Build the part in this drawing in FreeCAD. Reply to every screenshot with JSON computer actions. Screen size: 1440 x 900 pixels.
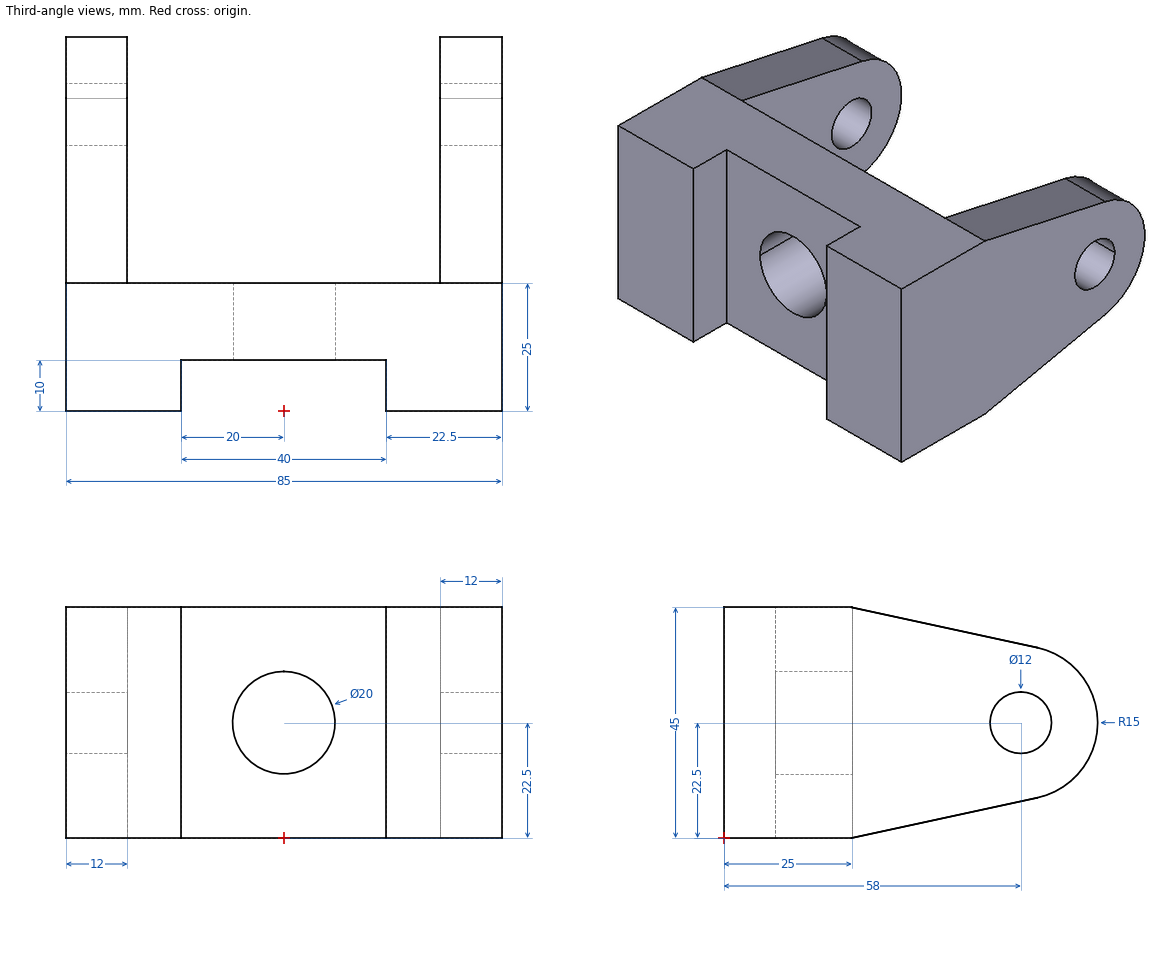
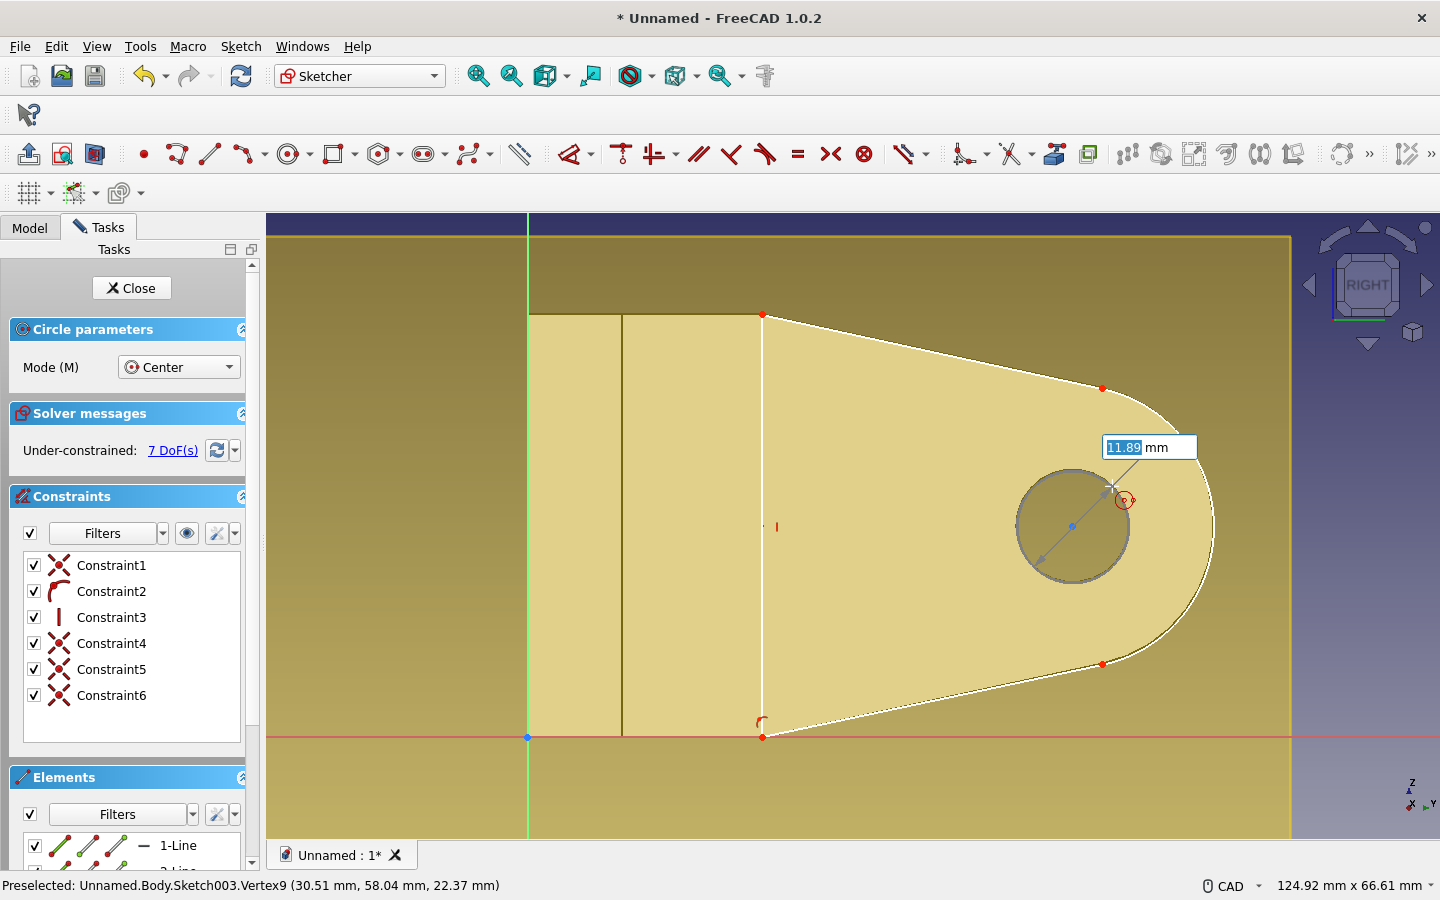
{"action": "type", "text": "12"}
{"action": "key", "text": "Return"}
{"action": "key", "text": "Escape"}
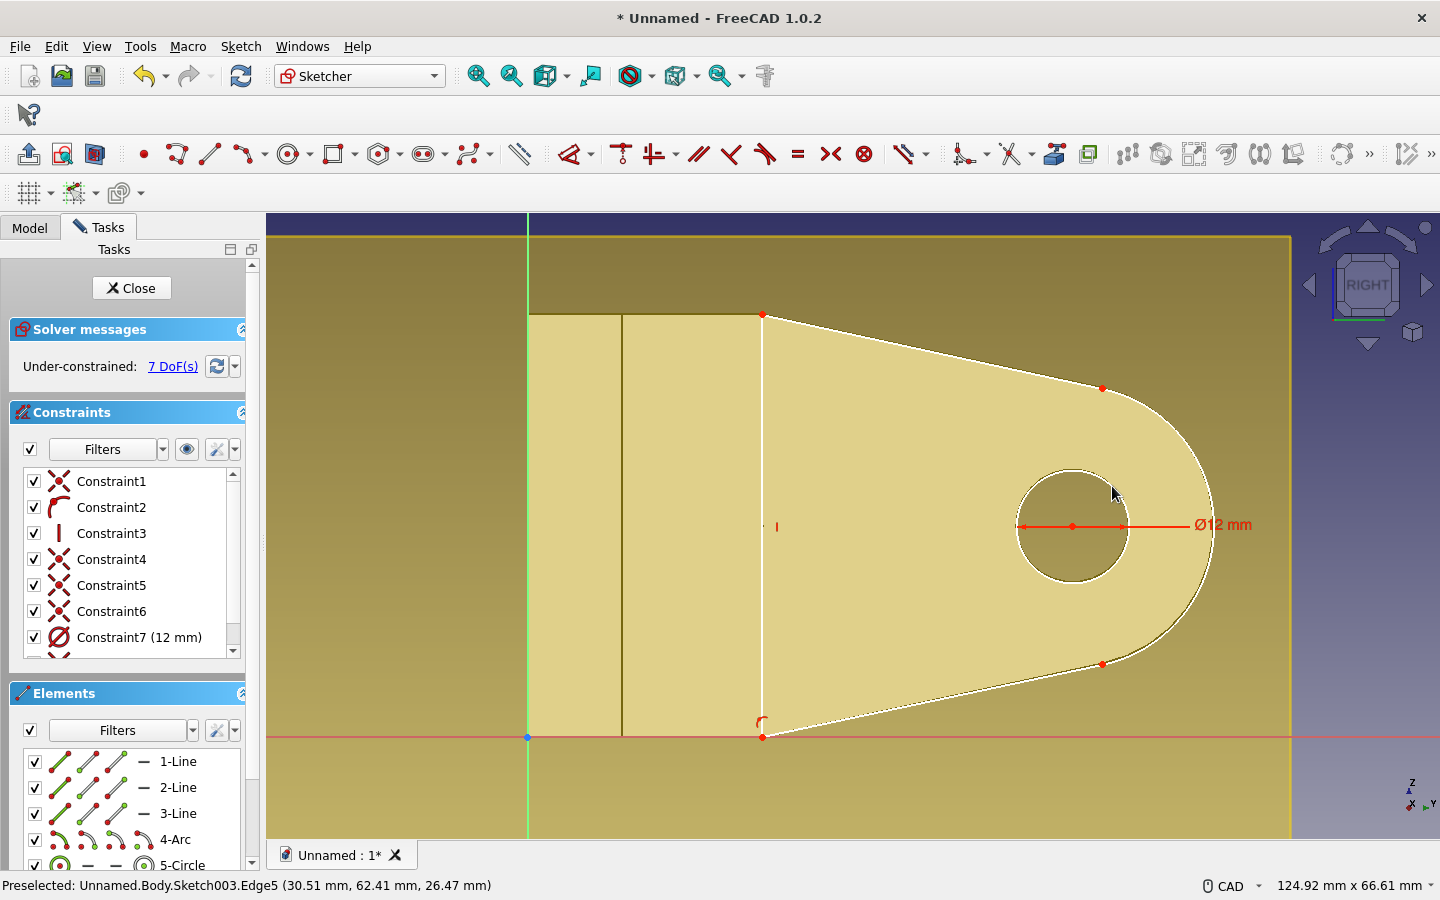
{"action": "left_click", "coordinate": [1000, 367]}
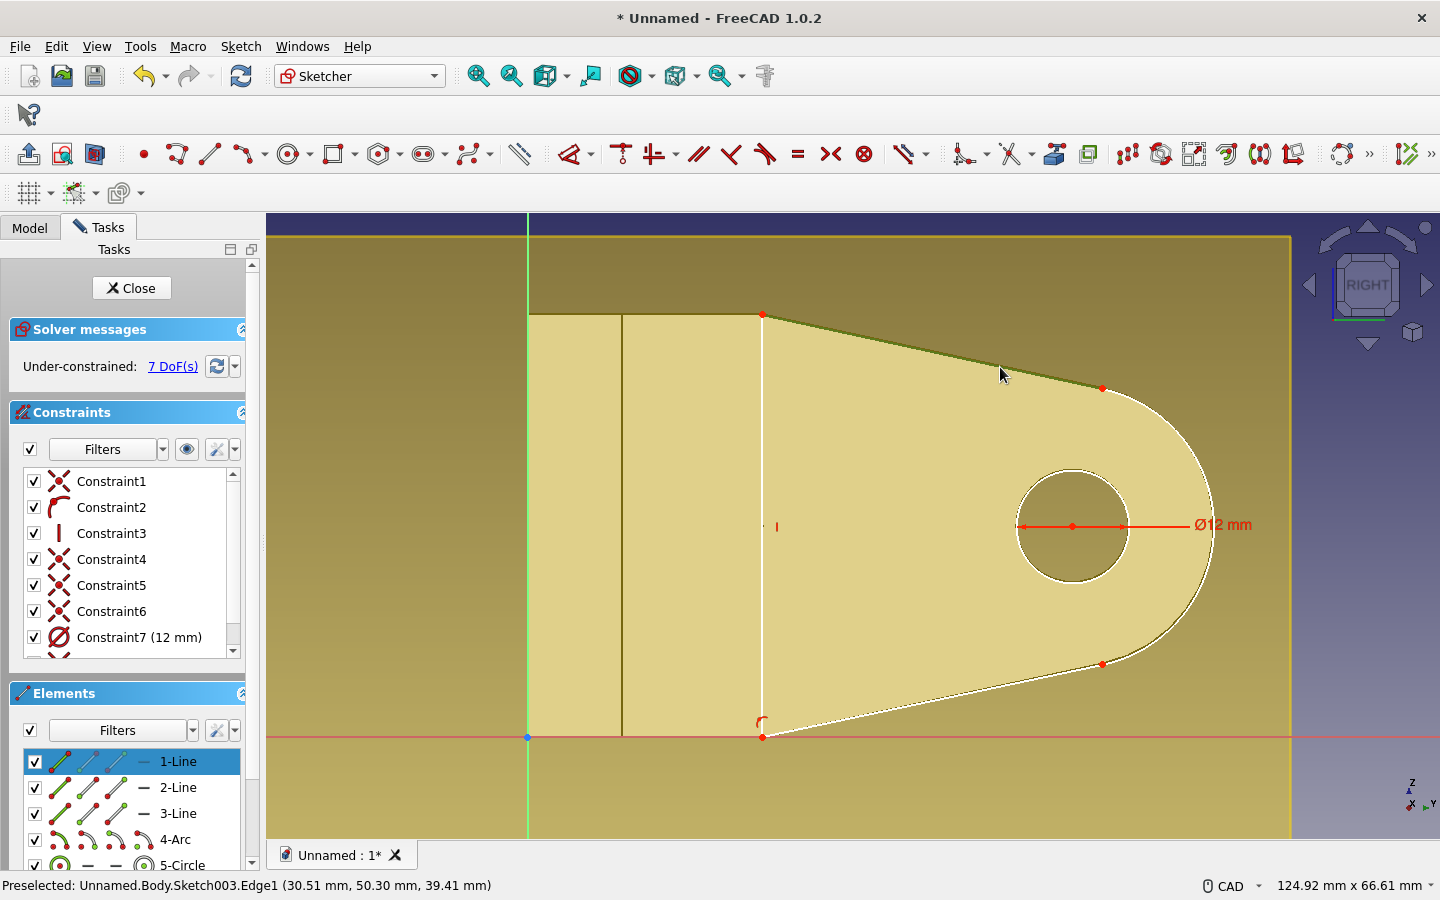
{"action": "left_click", "coordinate": [1194, 600]}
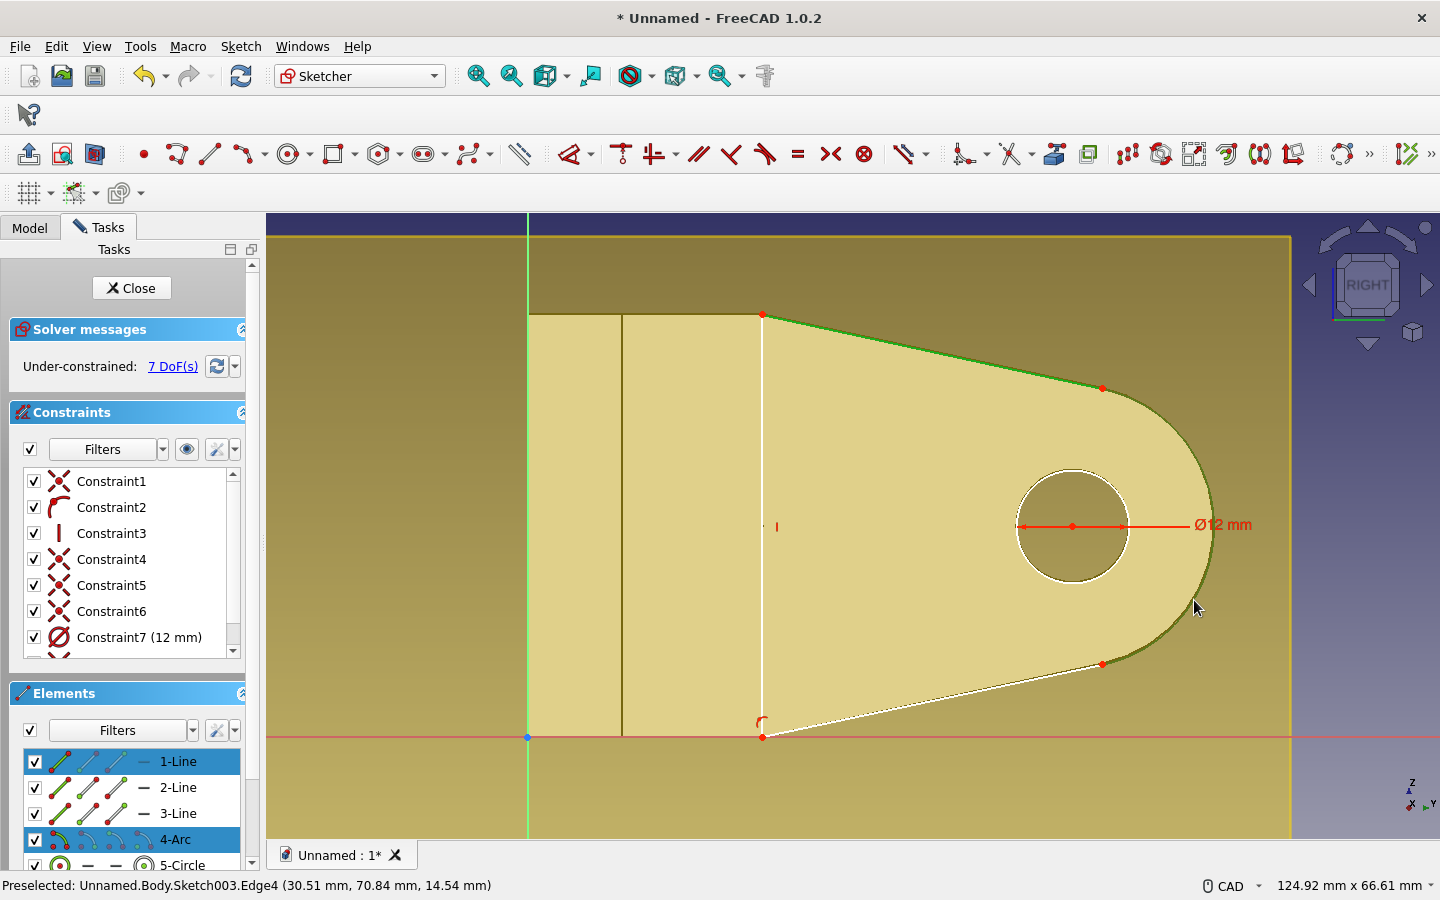
{"action": "left_click", "coordinate": [765, 154]}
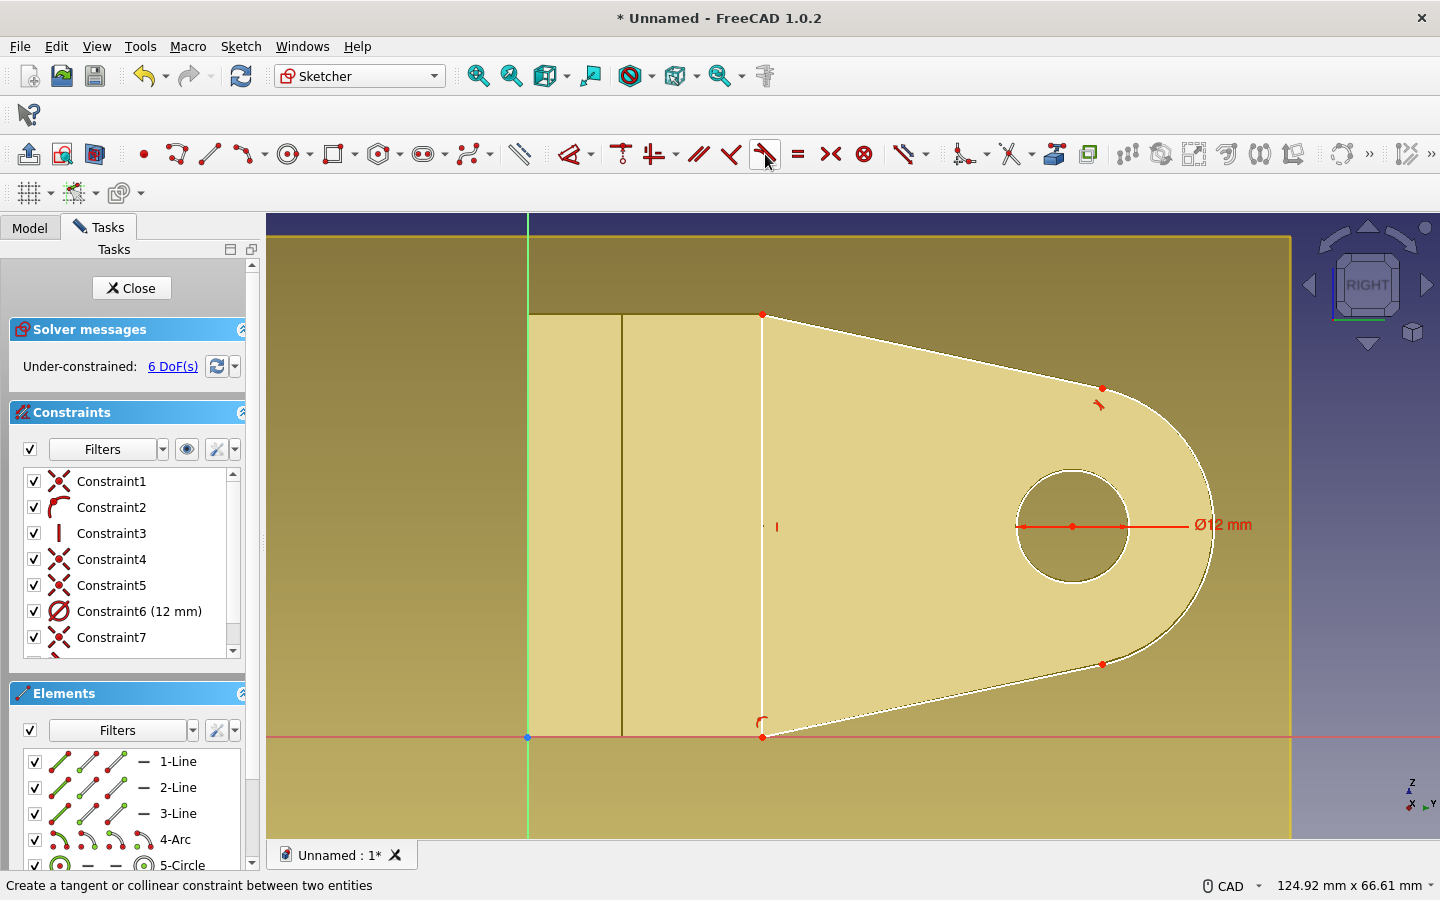
{"action": "left_click", "coordinate": [864, 716]}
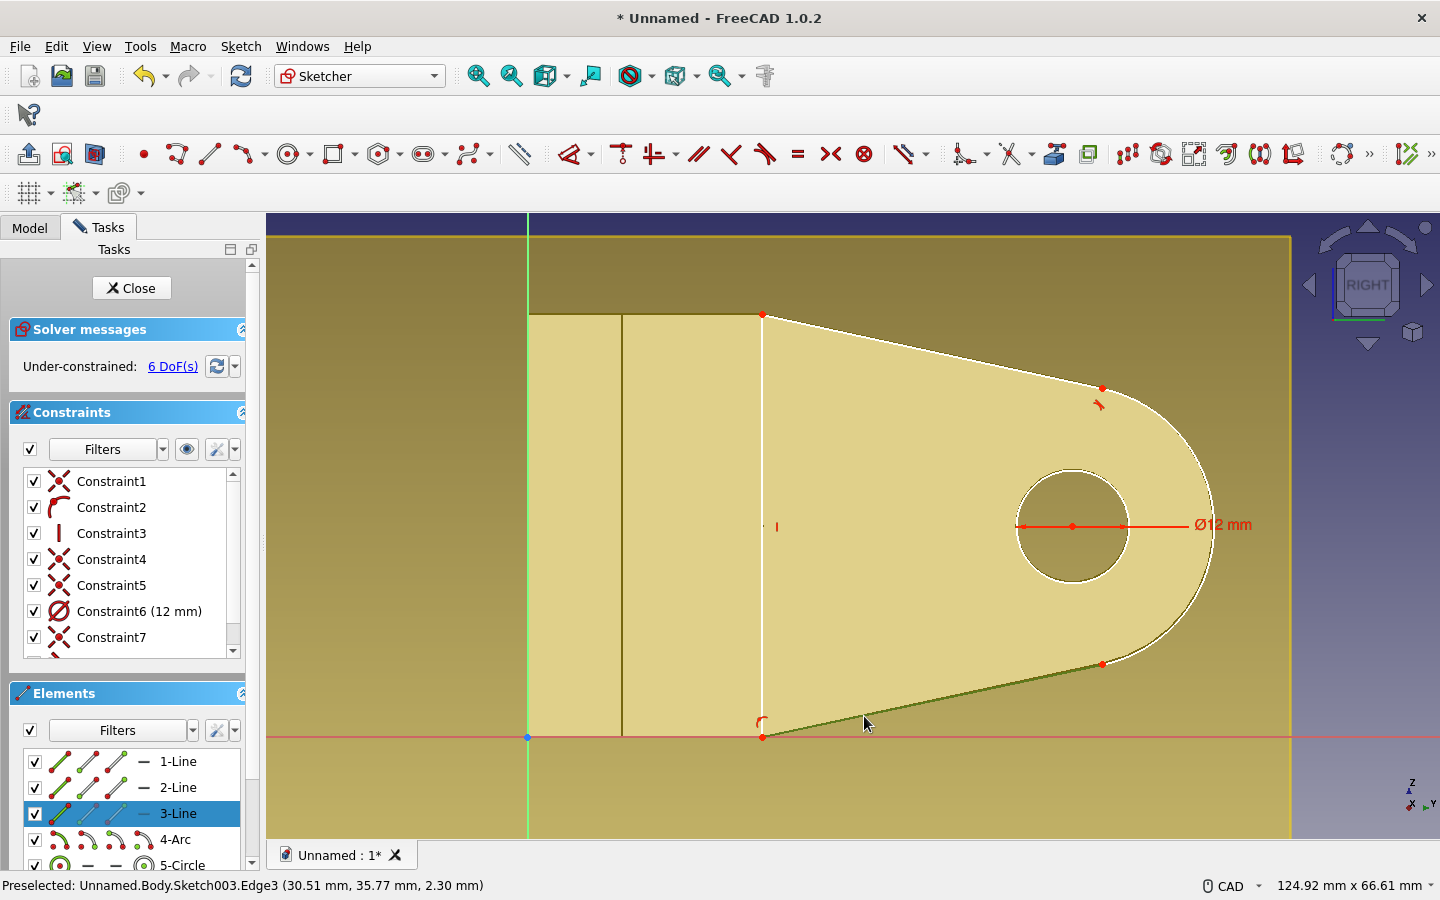
{"action": "left_click", "coordinate": [1193, 600]}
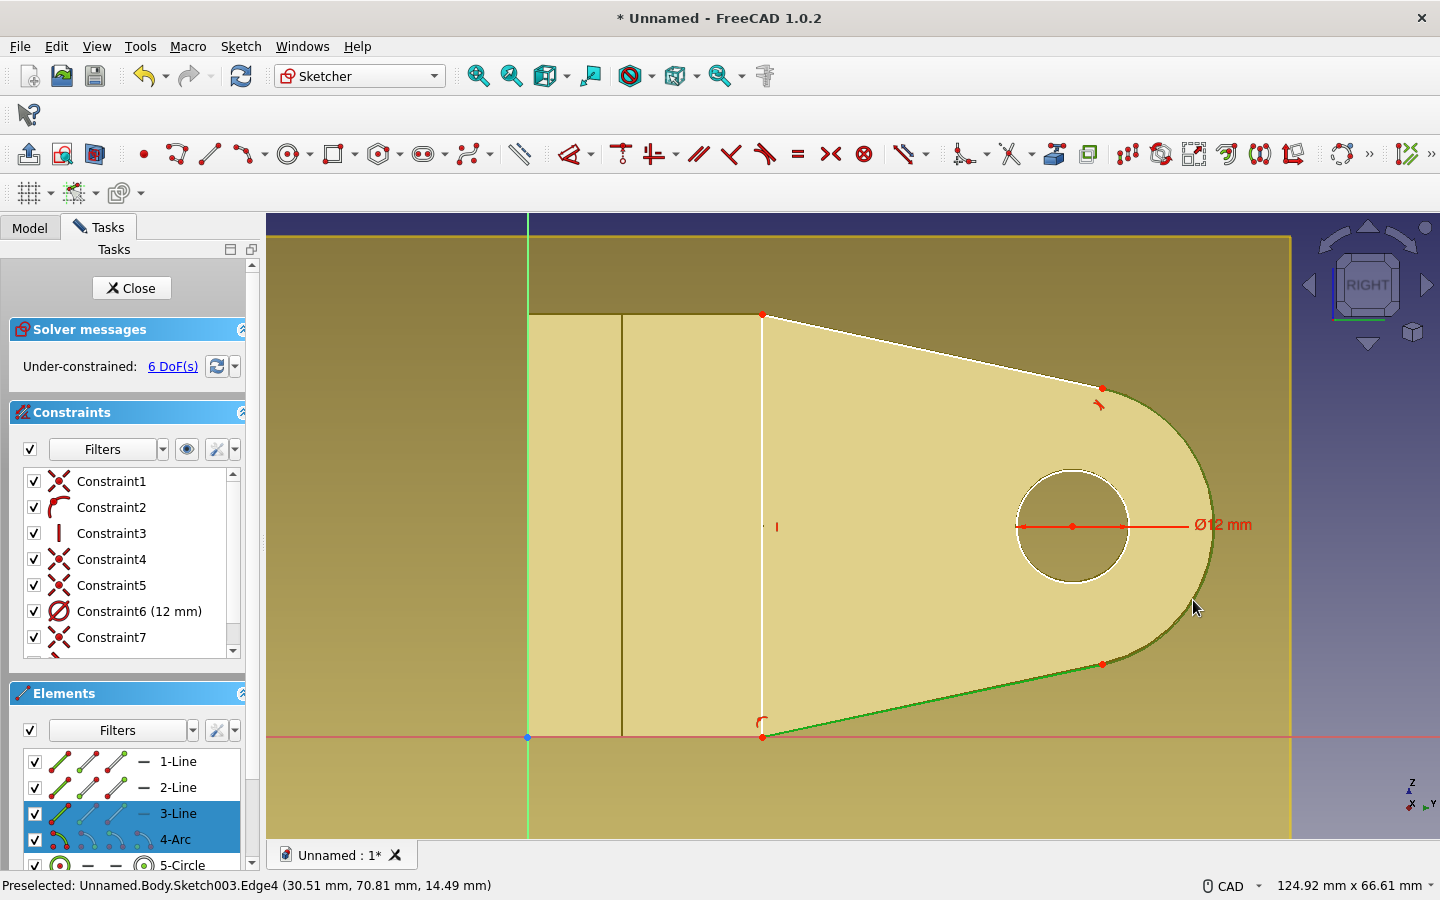
{"action": "left_click", "coordinate": [765, 154]}